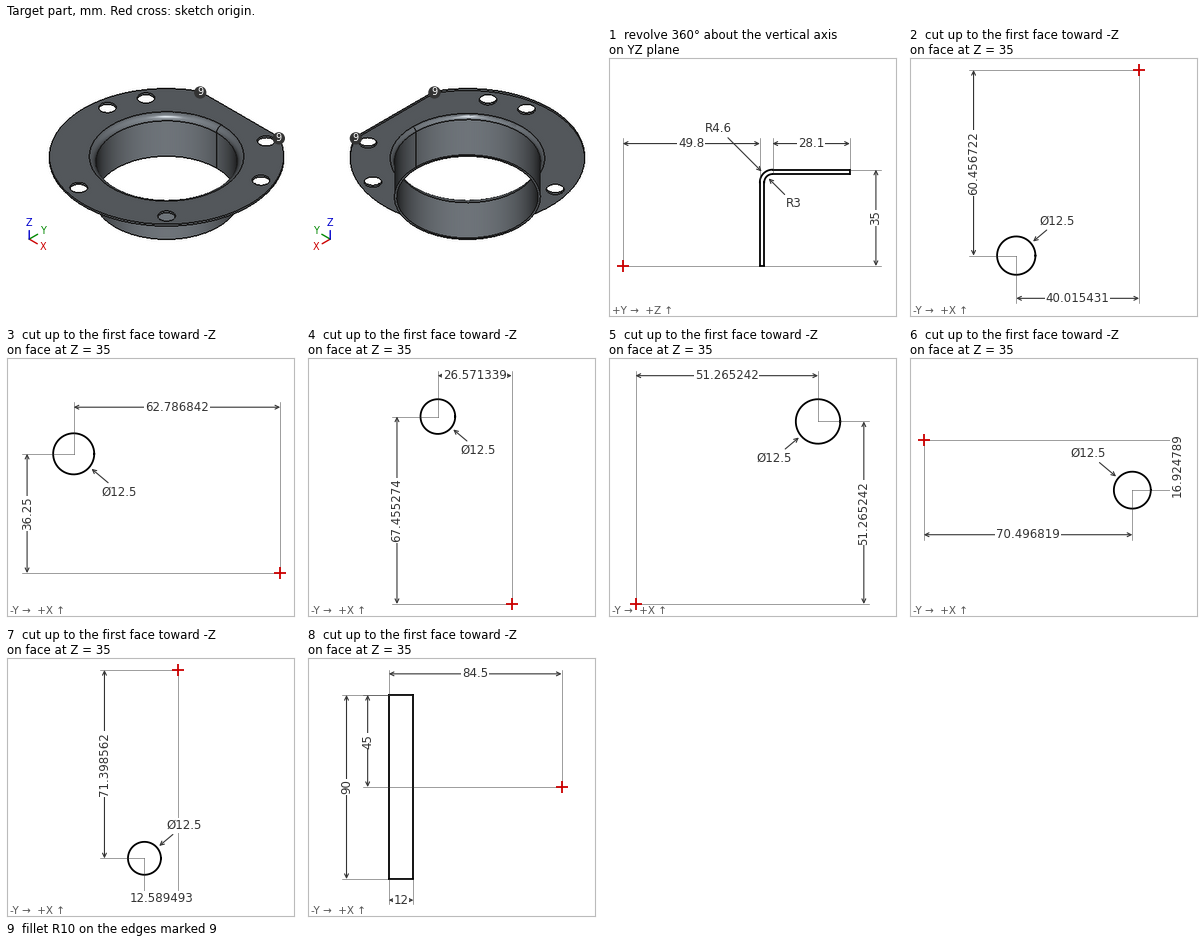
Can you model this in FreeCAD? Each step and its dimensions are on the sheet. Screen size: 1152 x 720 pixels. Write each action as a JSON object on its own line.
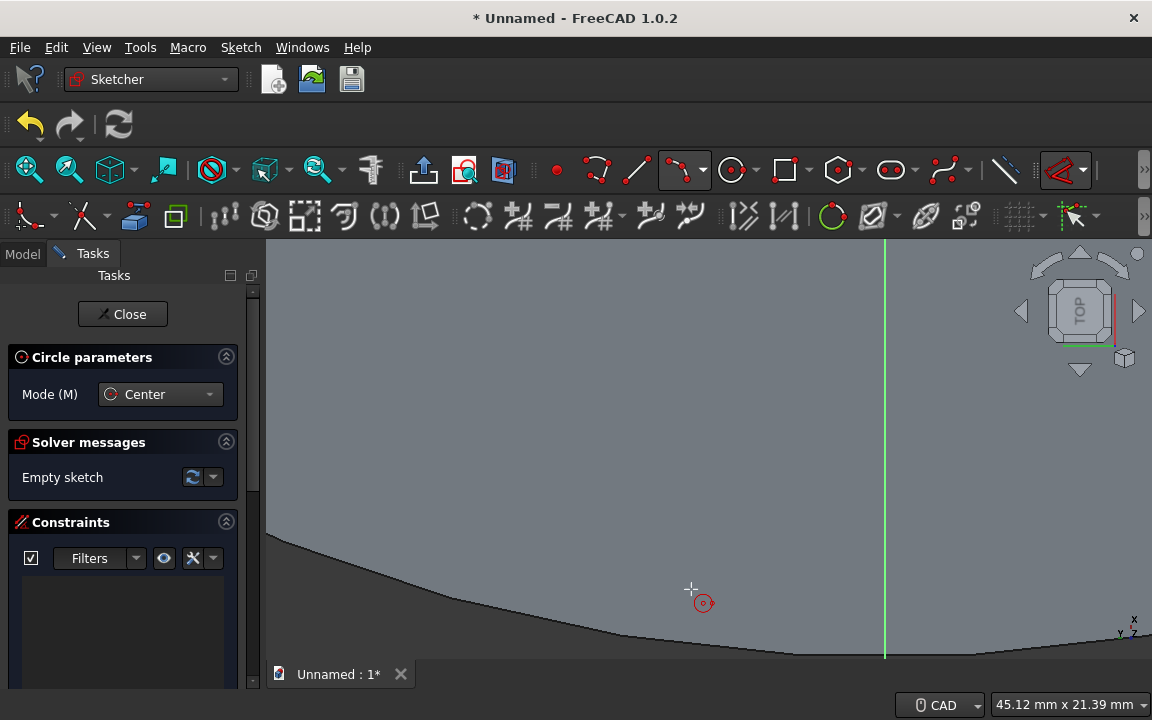
{"action": "left_click", "coordinate": [637, 439]}
{"action": "mouse_move", "coordinate": [724, 353]}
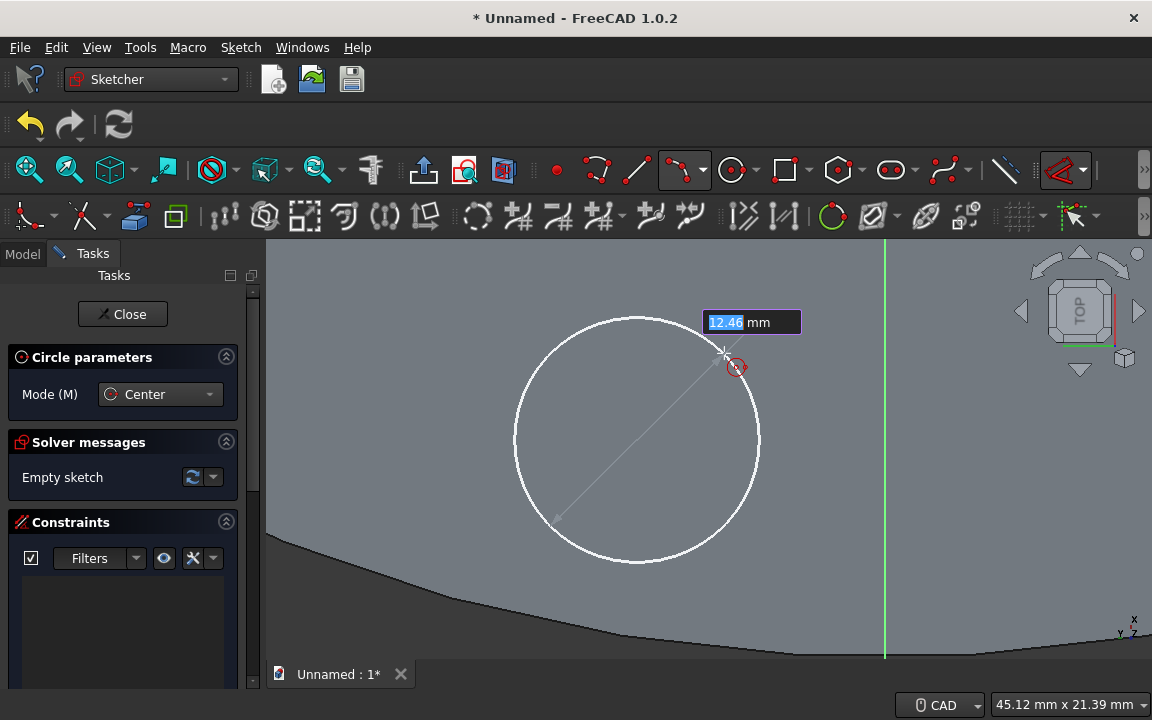
{"action": "type", "text": "12.5"}
{"action": "key", "text": "Return"}
{"action": "key", "text": "Escape"}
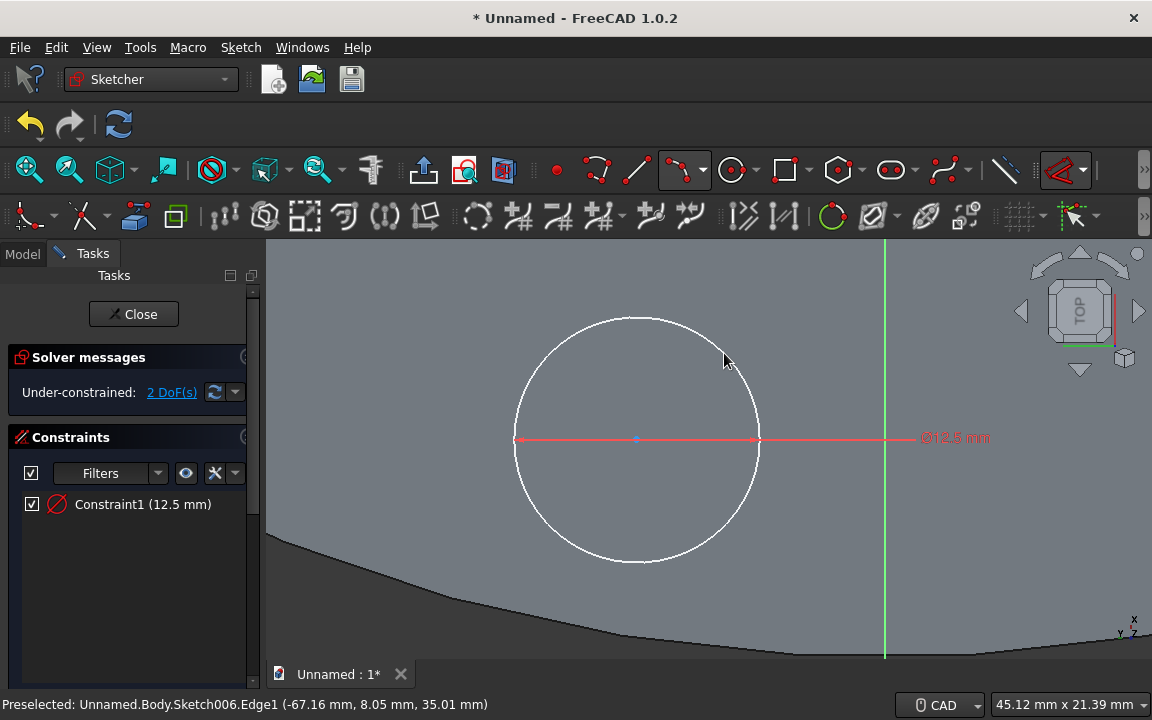
{"action": "left_click", "coordinate": [637, 440]}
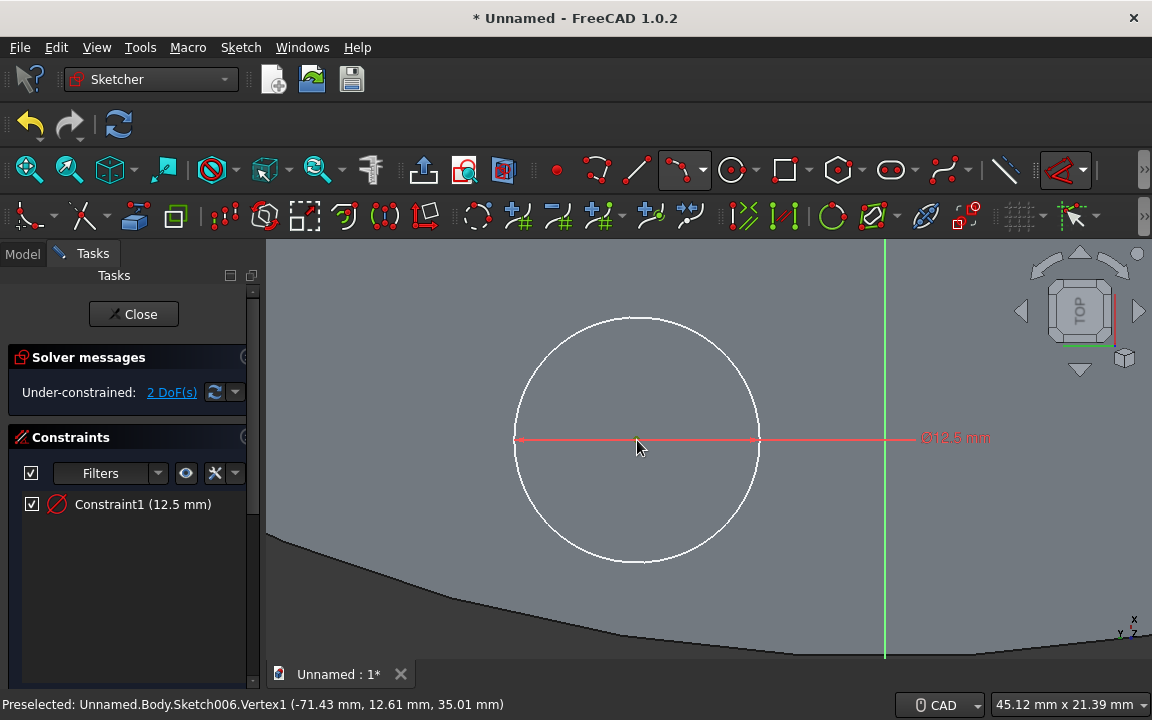
{"action": "key", "text": "l"}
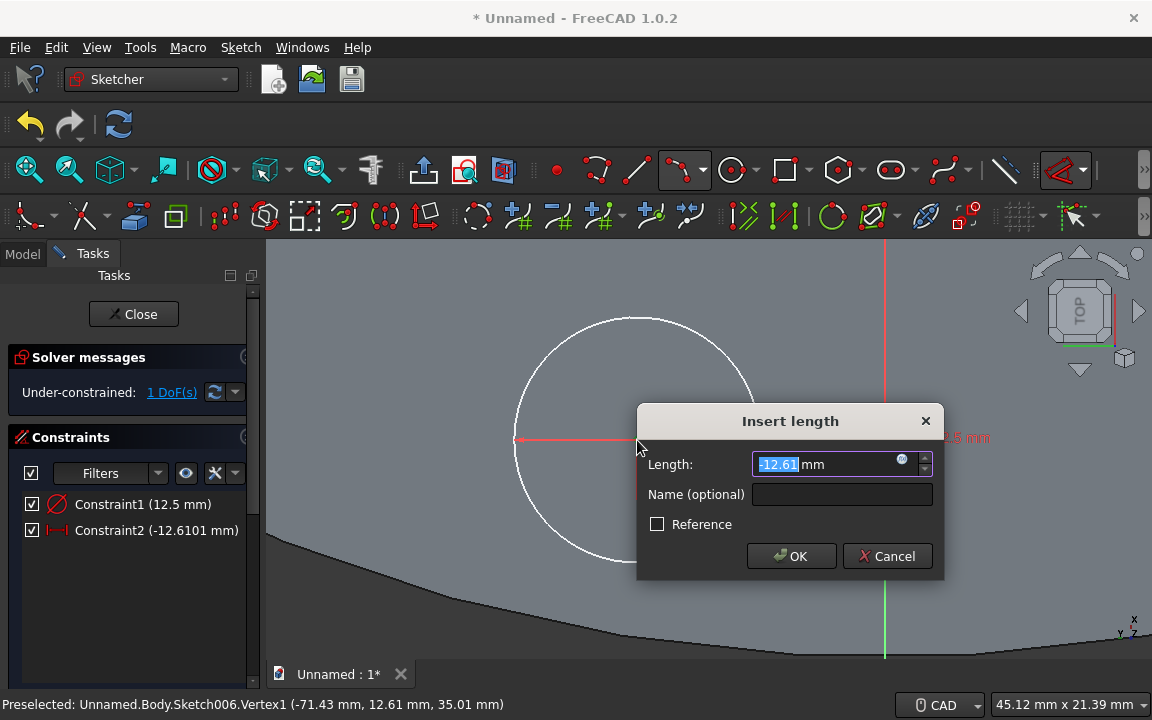
{"action": "type", "text": "-12.589493"}
{"action": "key", "text": "Return"}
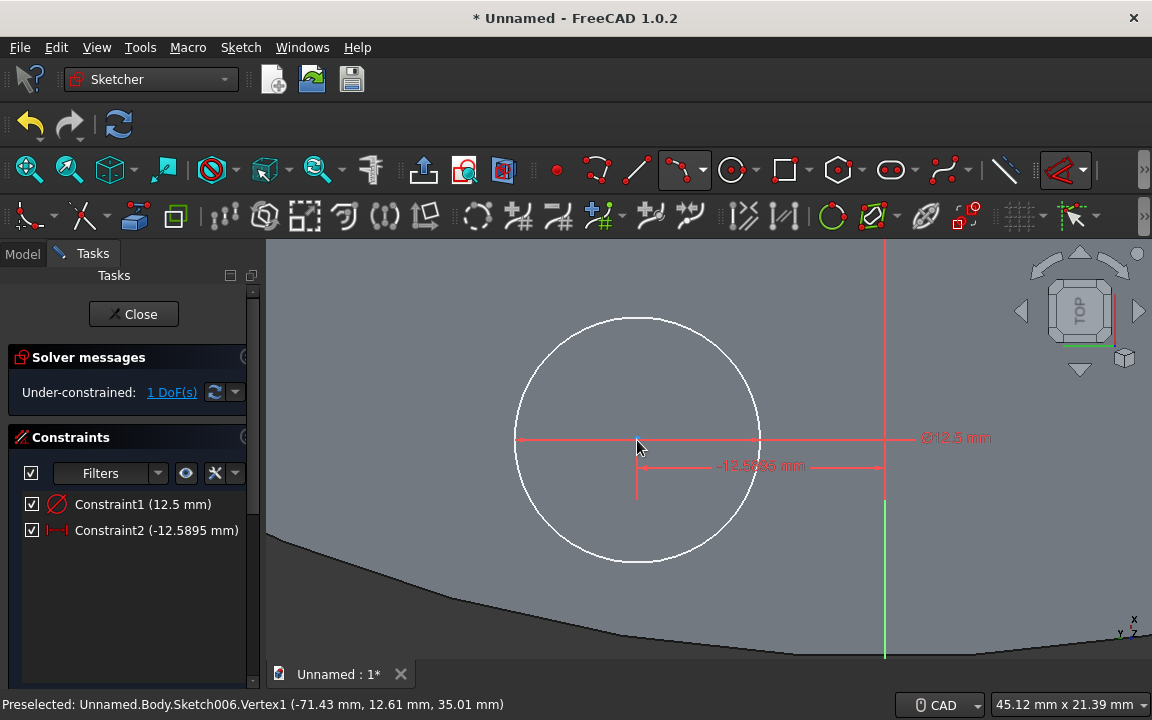
{"action": "left_click", "coordinate": [637, 440]}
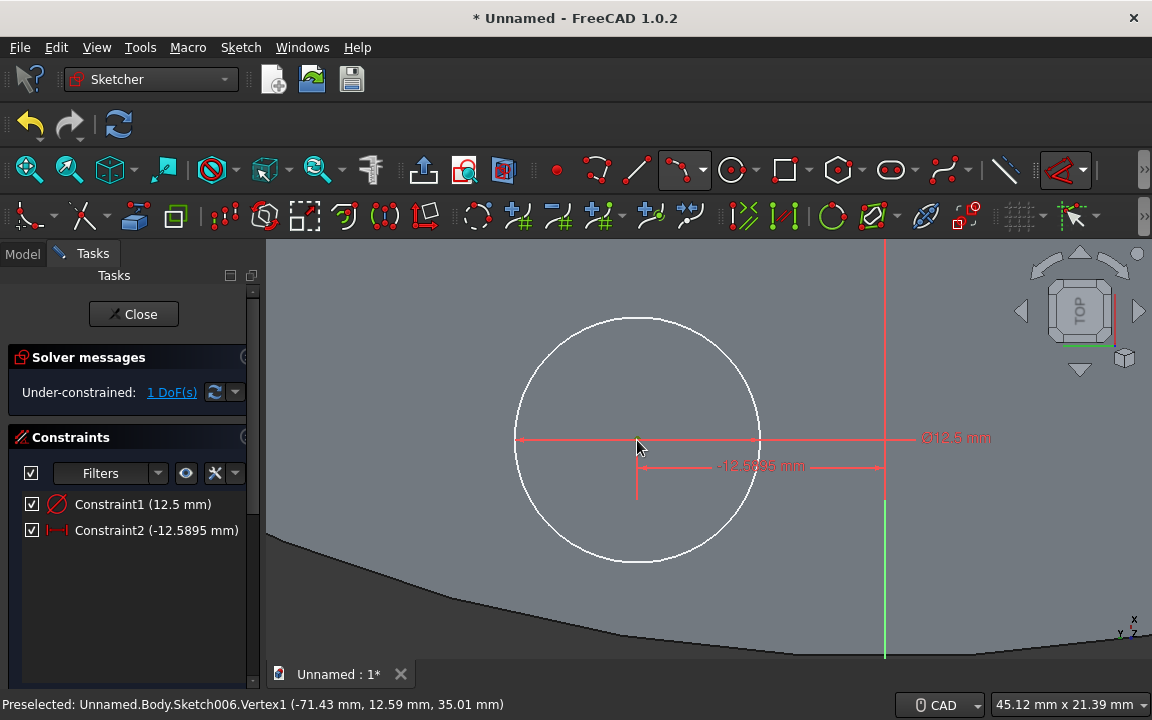
{"action": "key", "text": "i"}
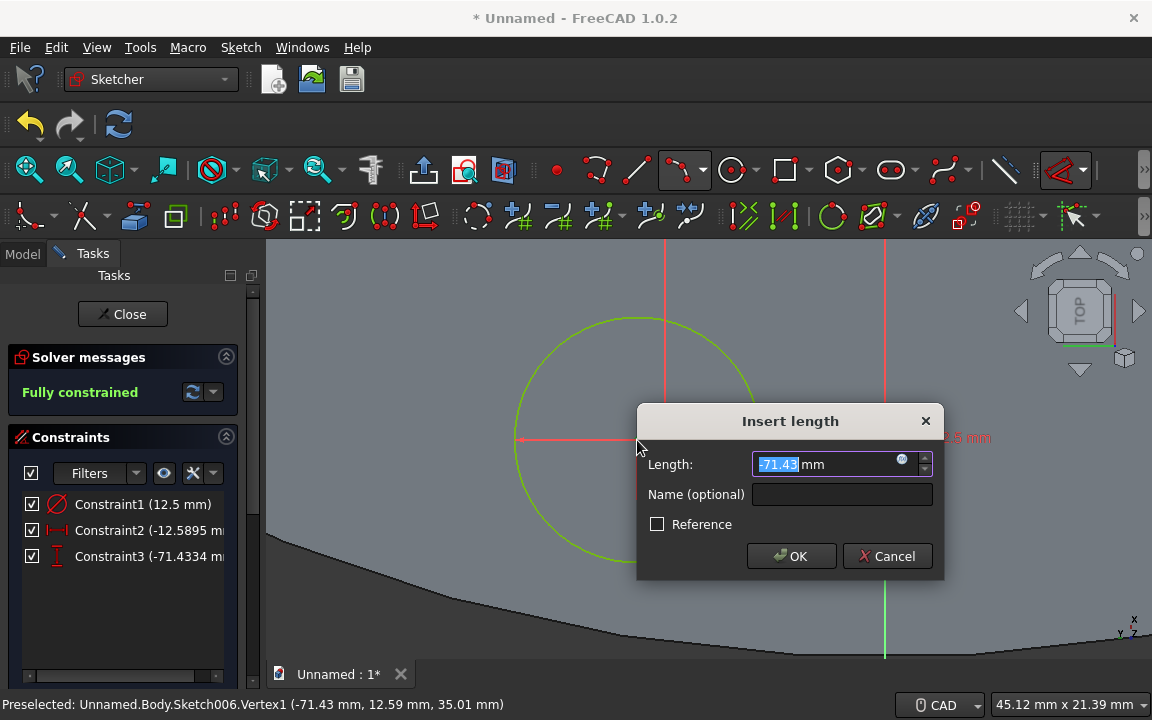
{"action": "type", "text": "-71.398562"}
{"action": "key", "text": "Return"}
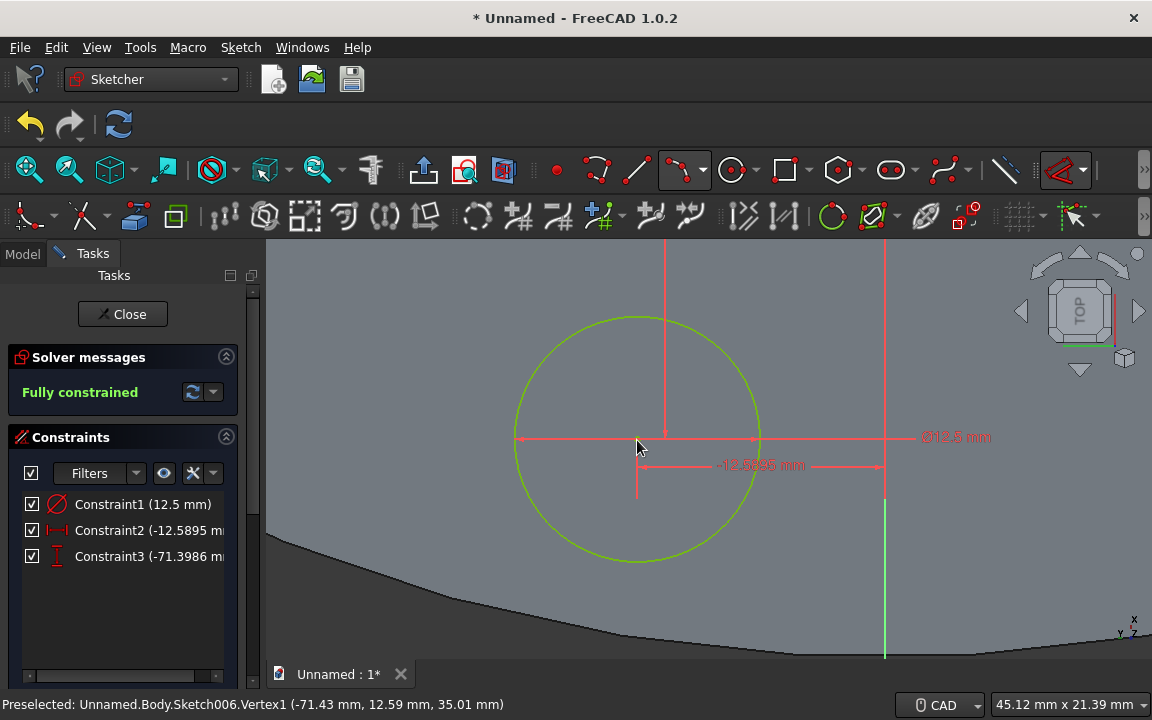
{"action": "left_click", "coordinate": [123, 314]}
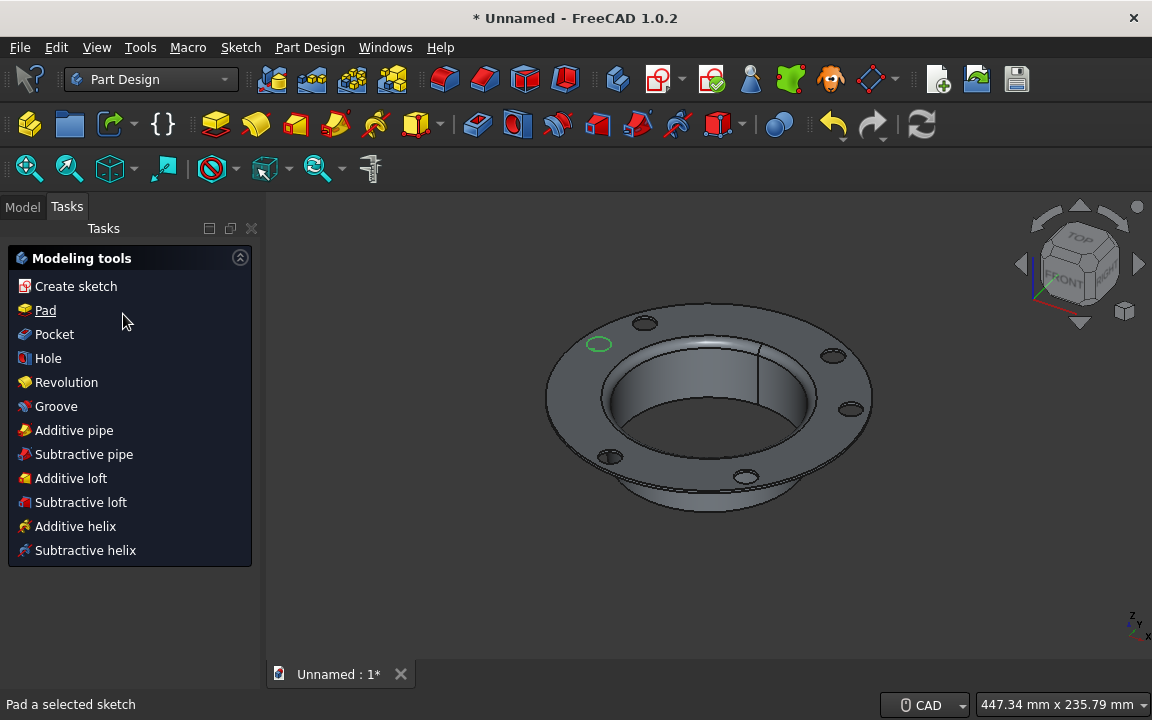
{"action": "left_click", "coordinate": [478, 124]}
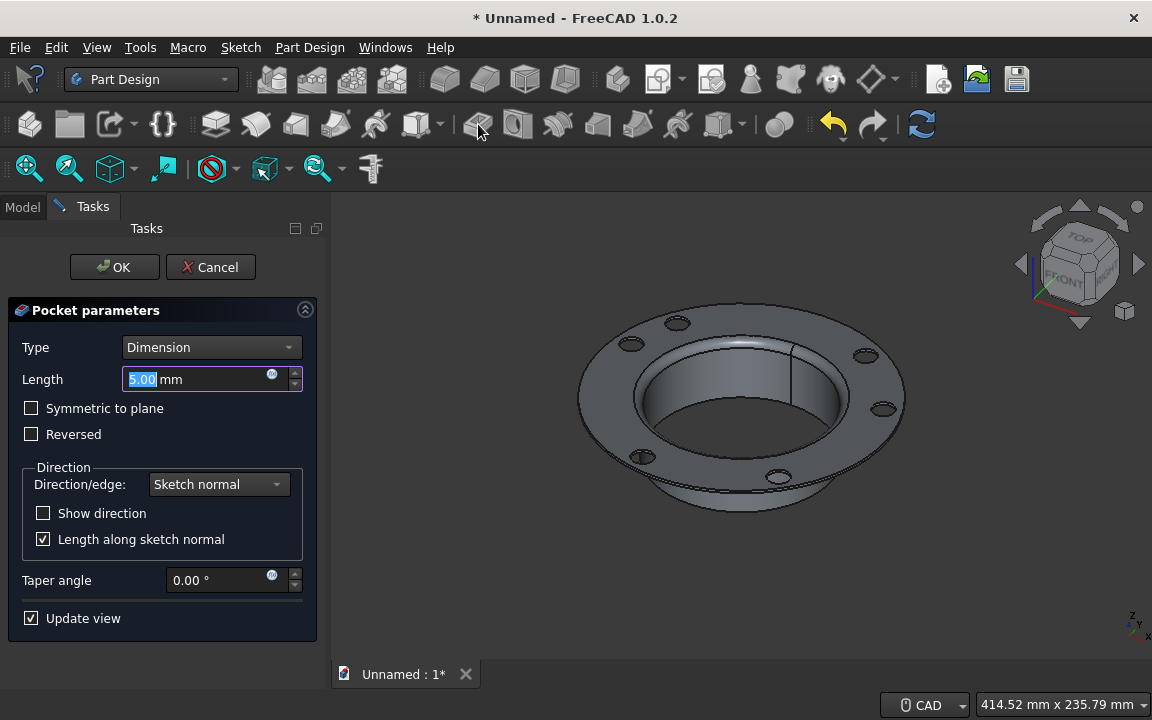
{"action": "left_click", "coordinate": [212, 348]}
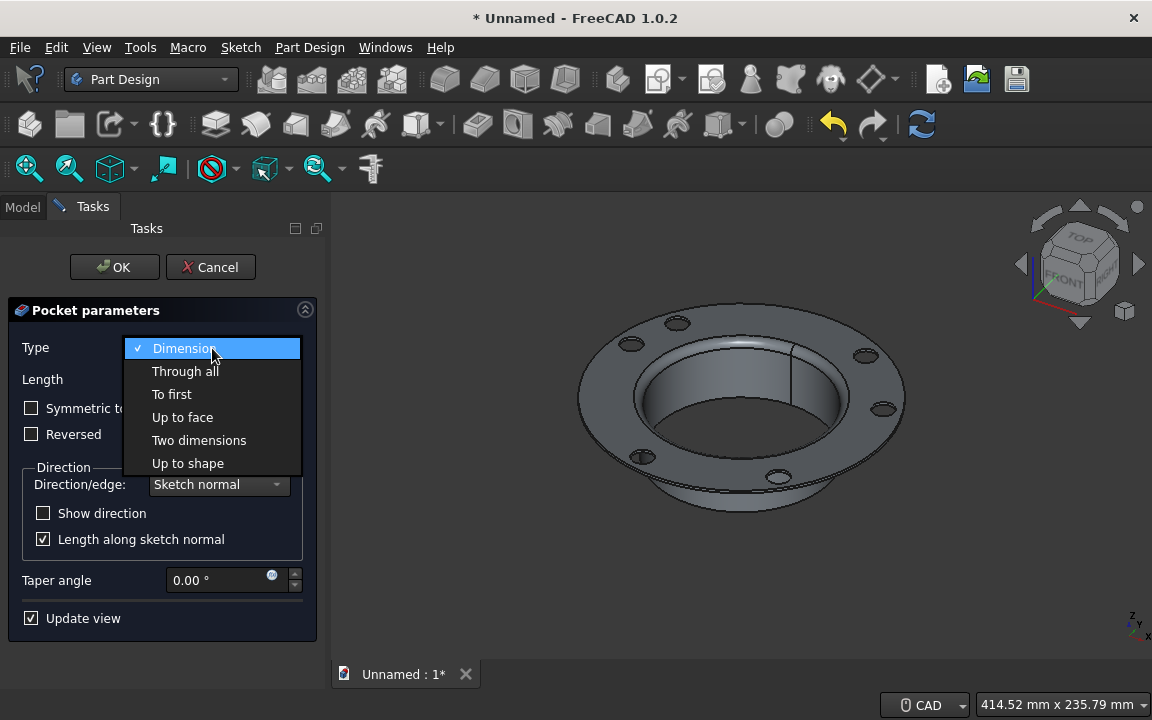
{"action": "left_click", "coordinate": [212, 394]}